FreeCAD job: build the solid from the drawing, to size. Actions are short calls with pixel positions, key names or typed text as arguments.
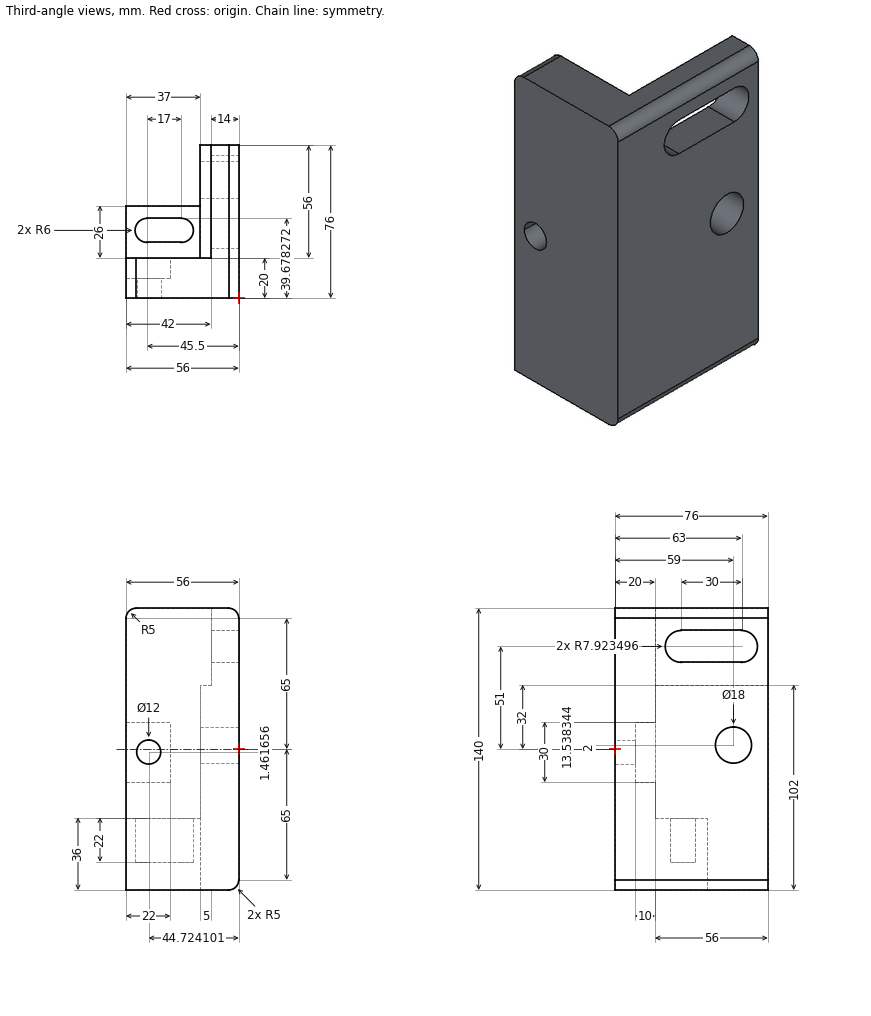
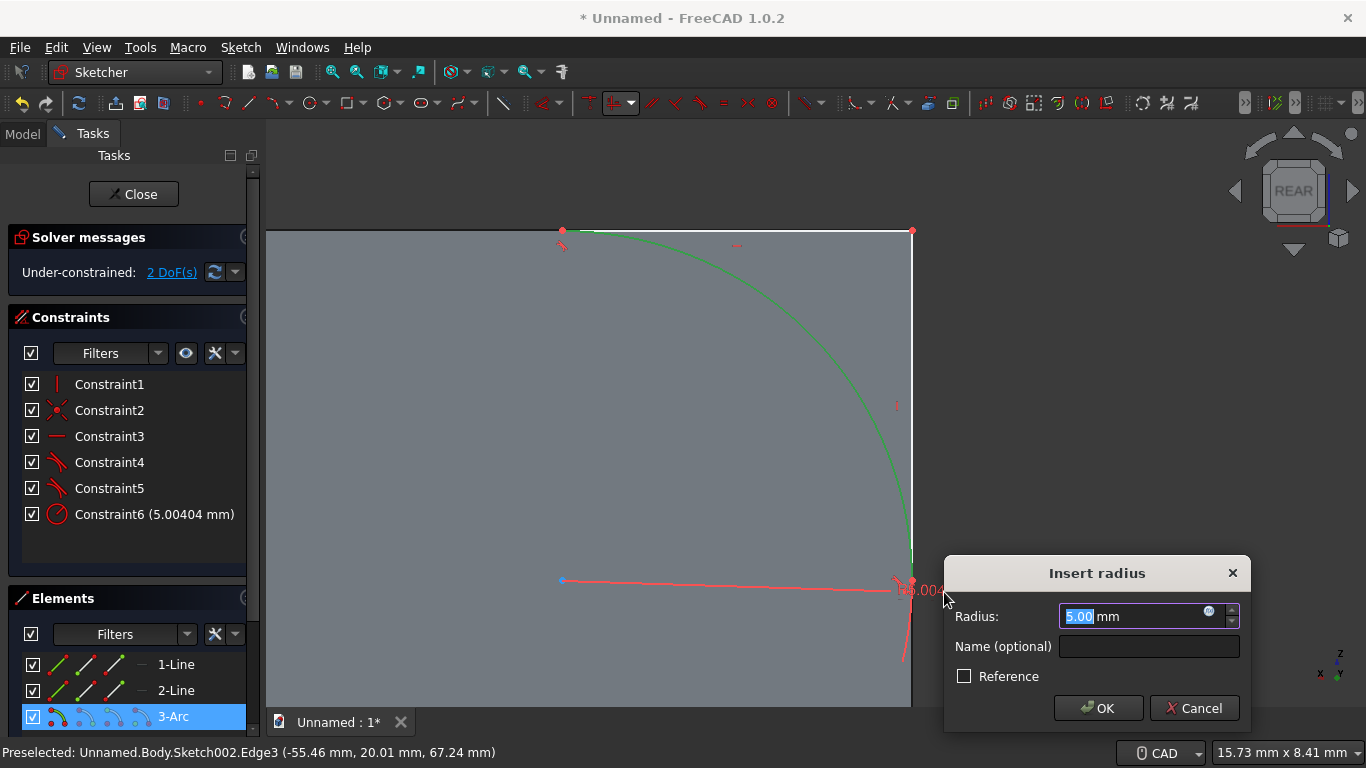
text(5)
key(Return)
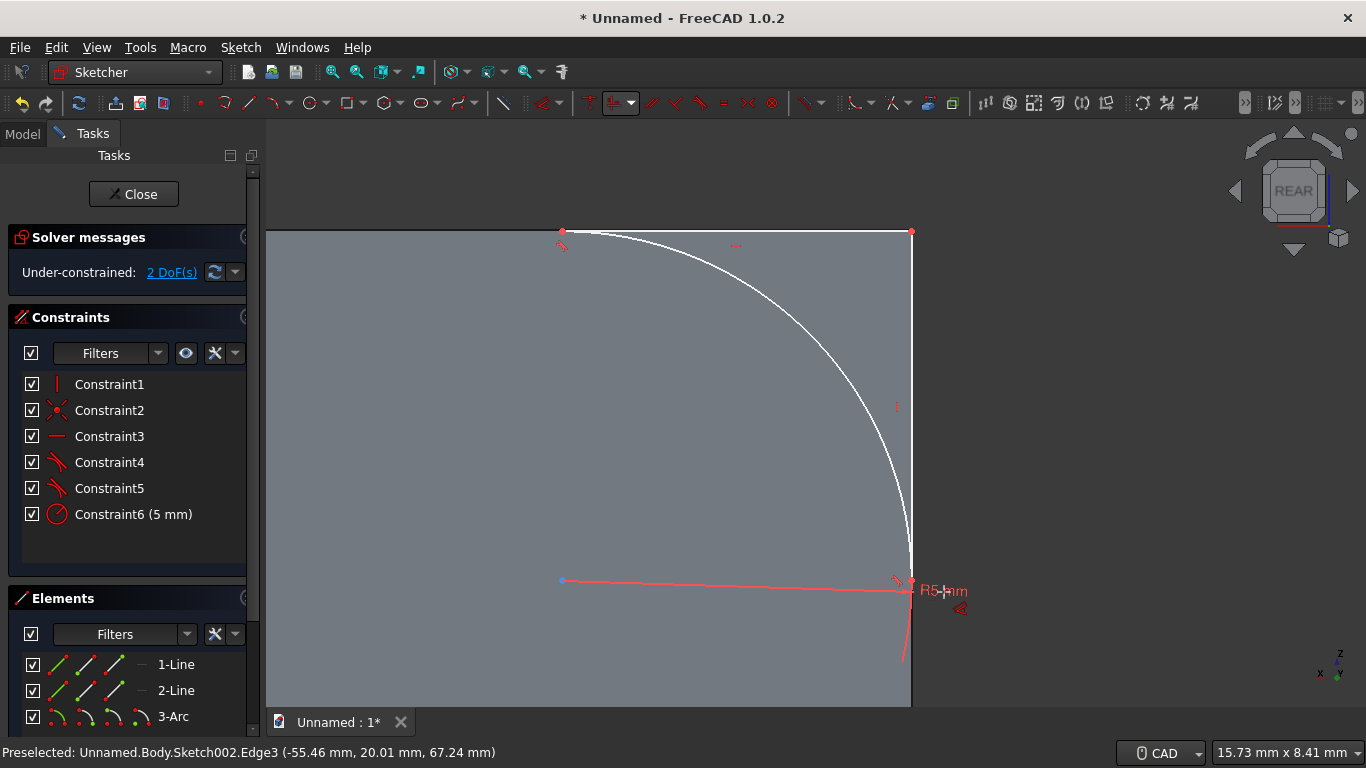
click(912, 581)
click(603, 547)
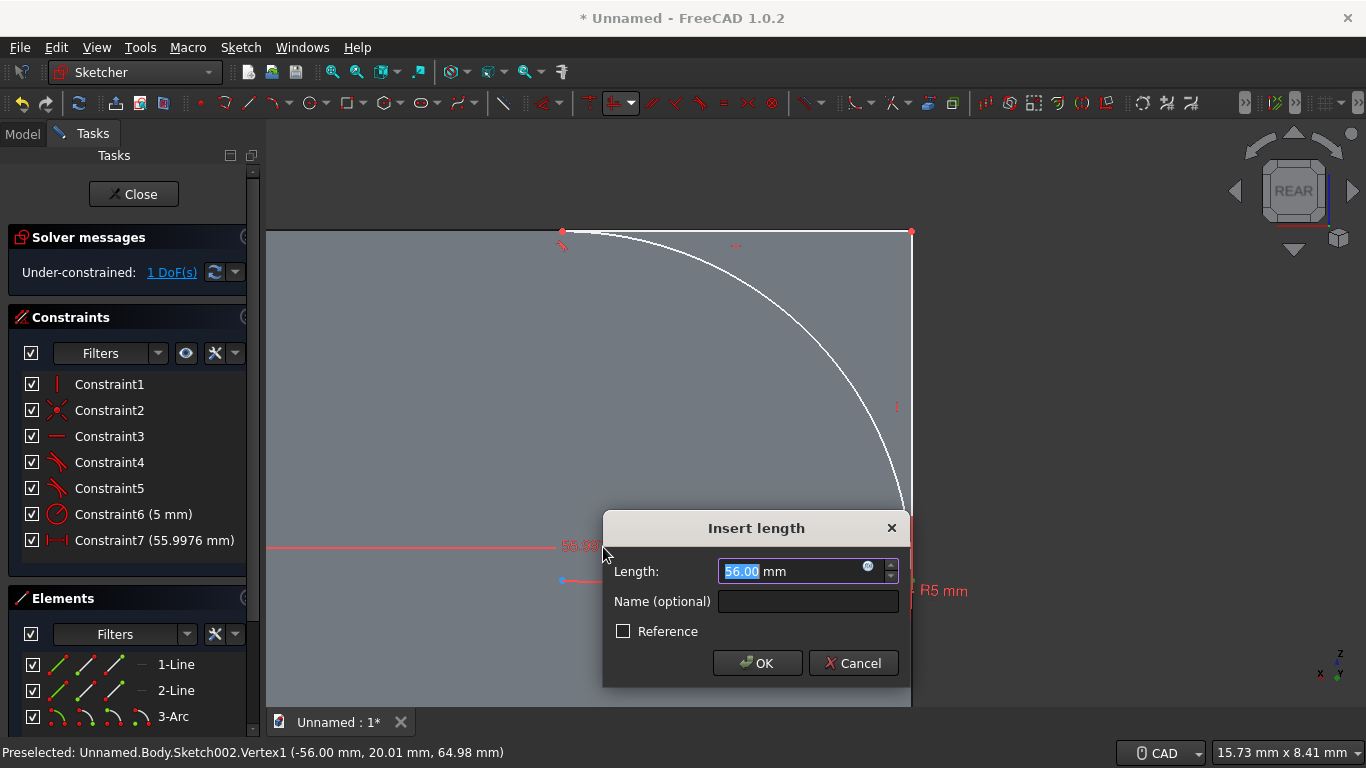
text(56)
key(Return)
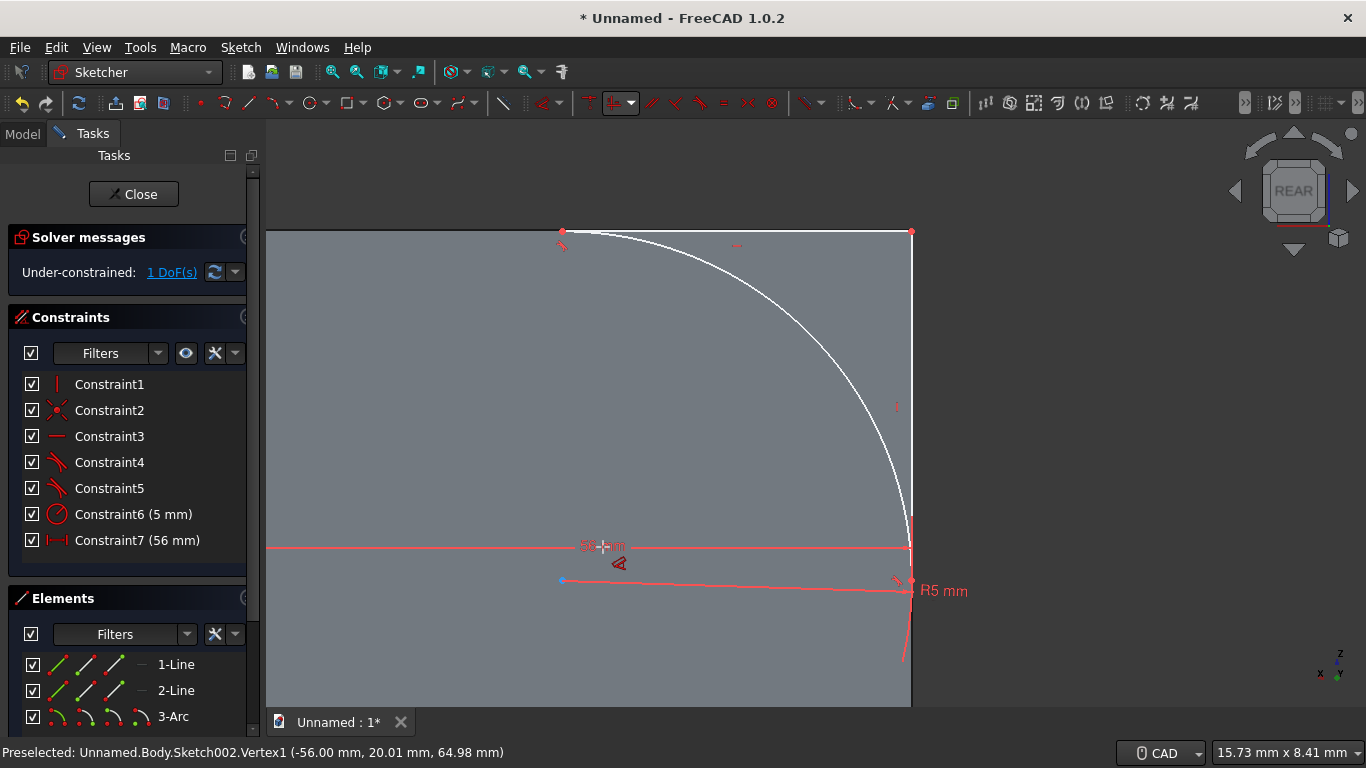
click(912, 581)
click(946, 630)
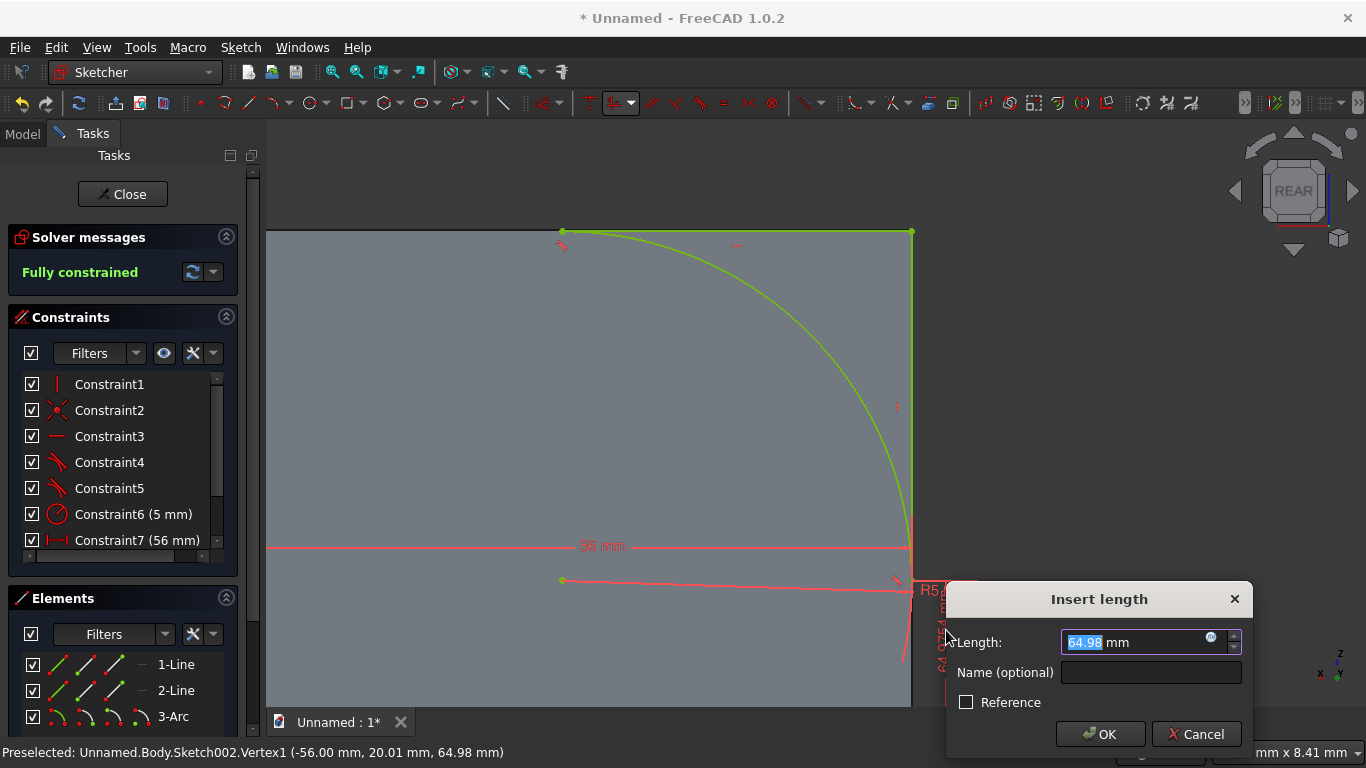
text(65)
key(Return)
key(Escape)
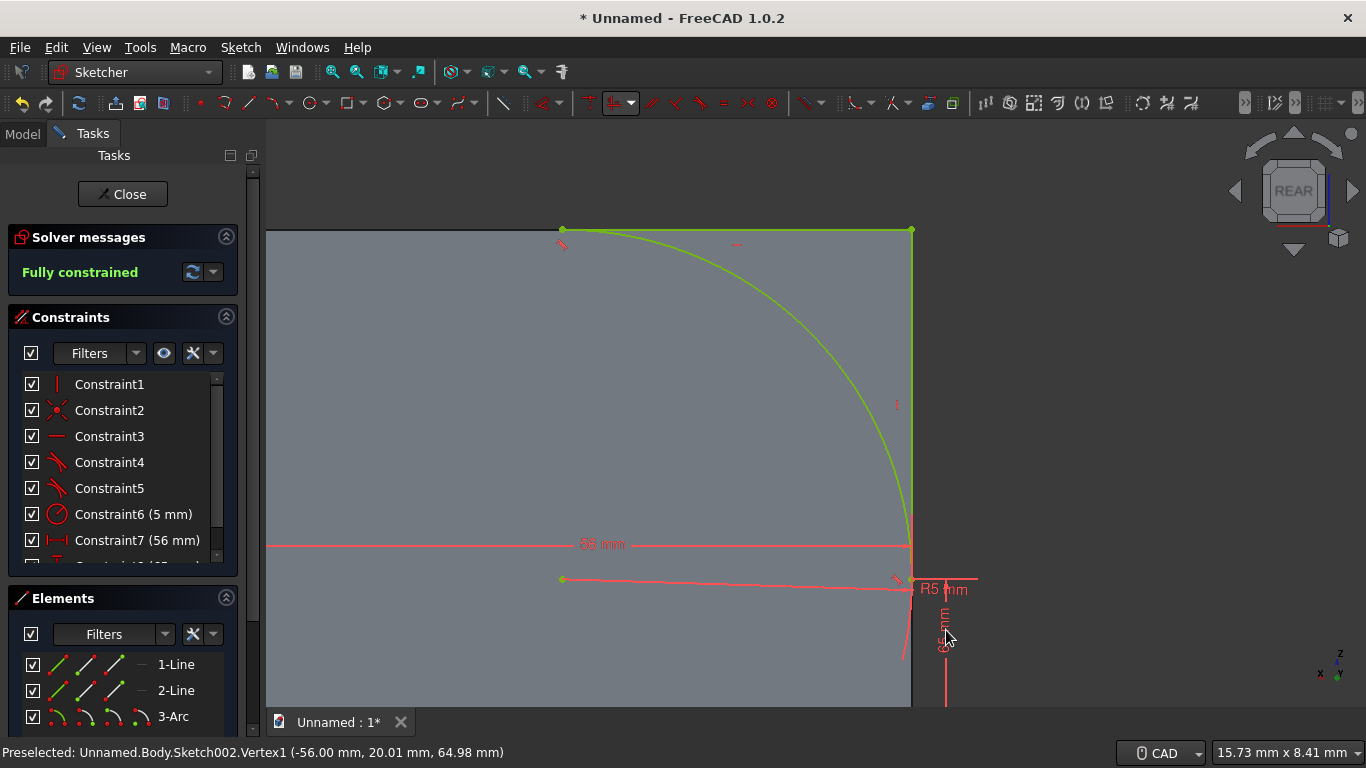
click(123, 194)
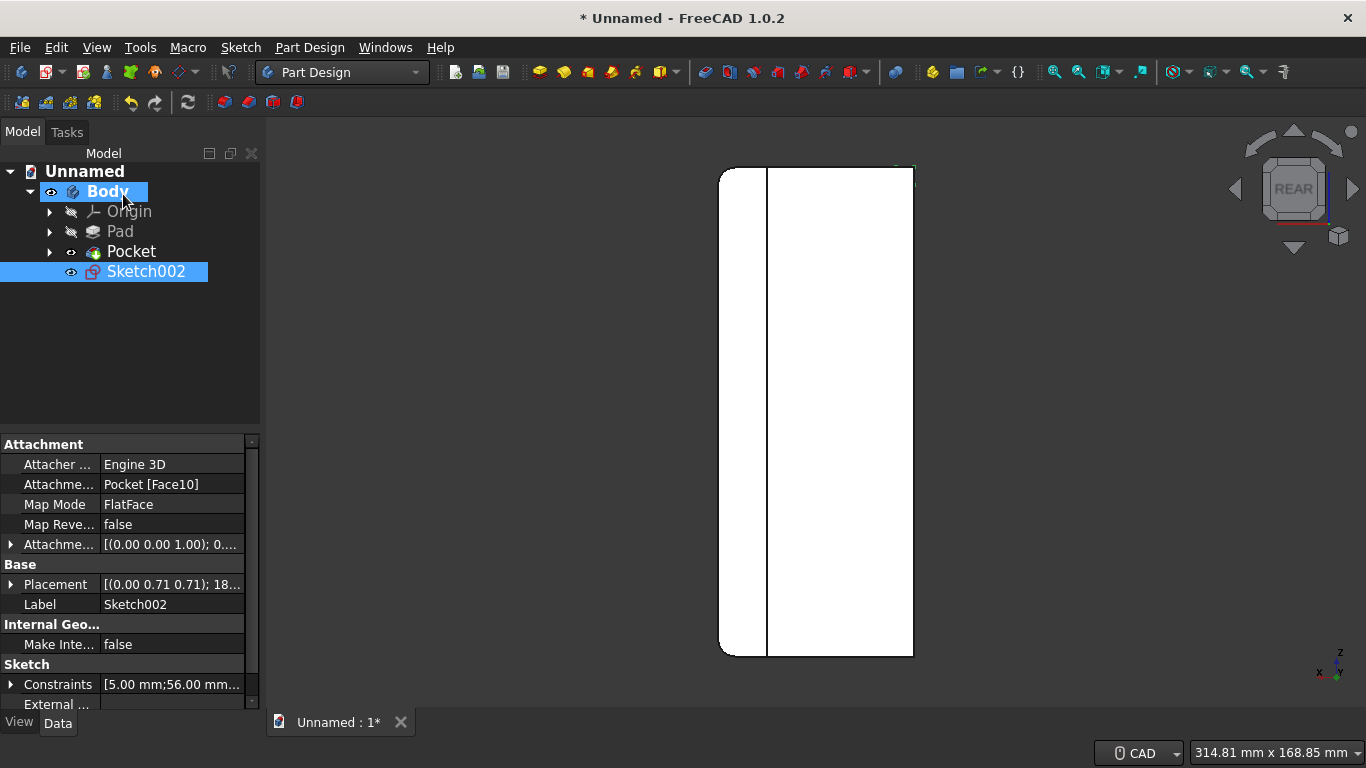
click(706, 72)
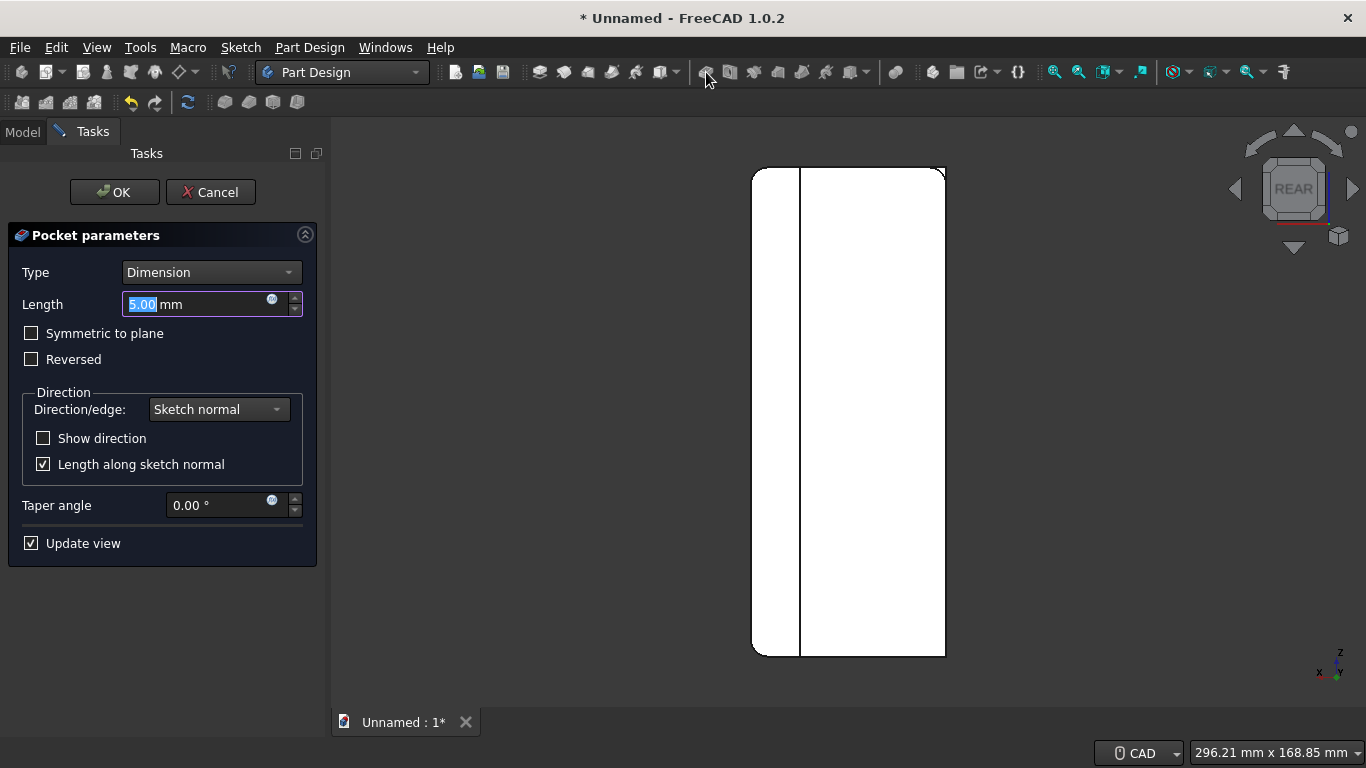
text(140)
key(Tab)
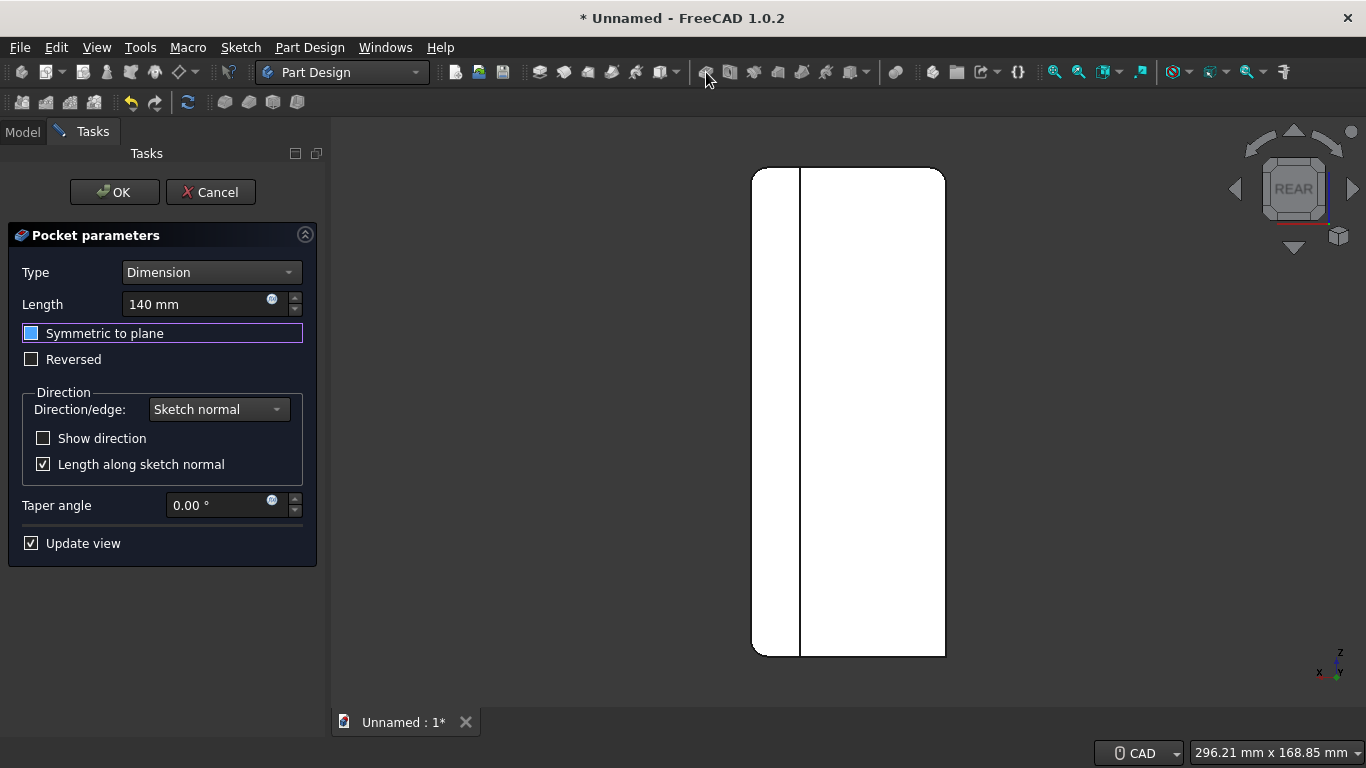
click(115, 192)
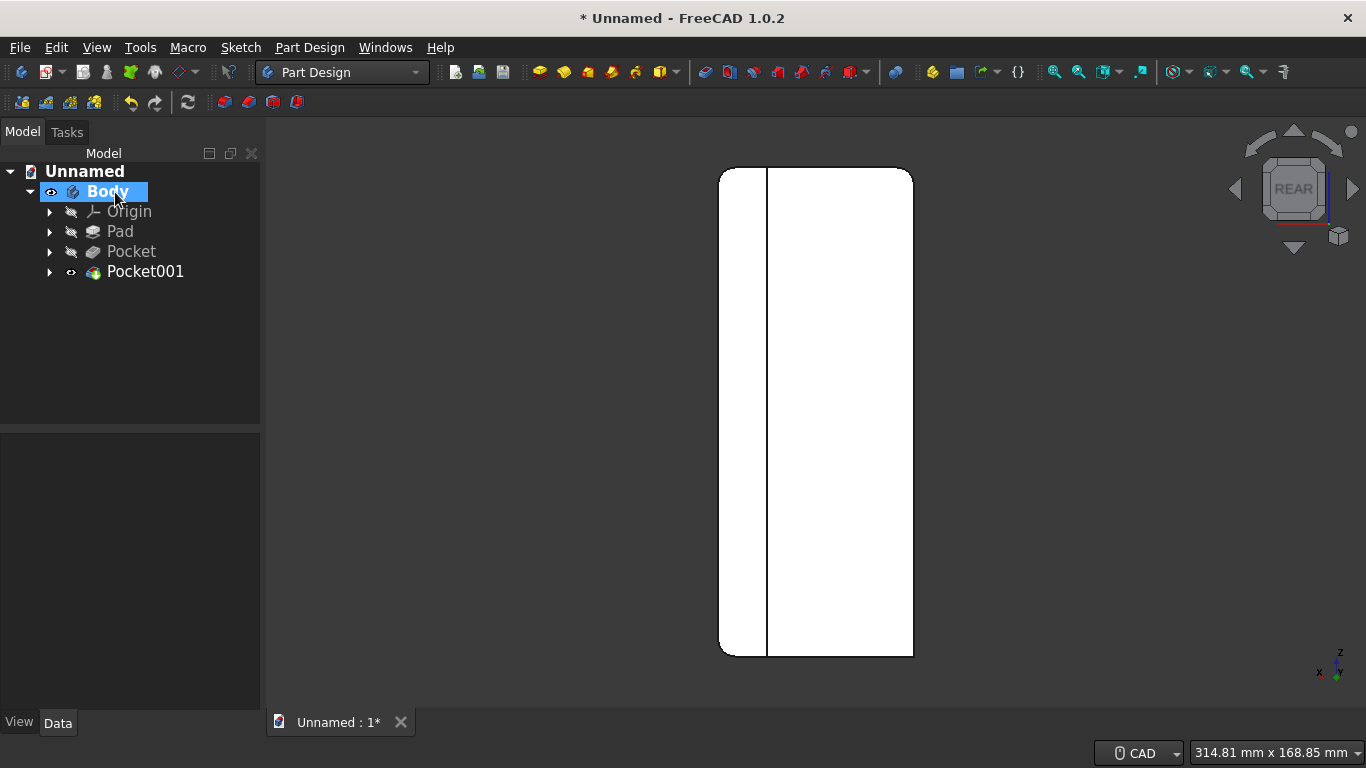
key(6)